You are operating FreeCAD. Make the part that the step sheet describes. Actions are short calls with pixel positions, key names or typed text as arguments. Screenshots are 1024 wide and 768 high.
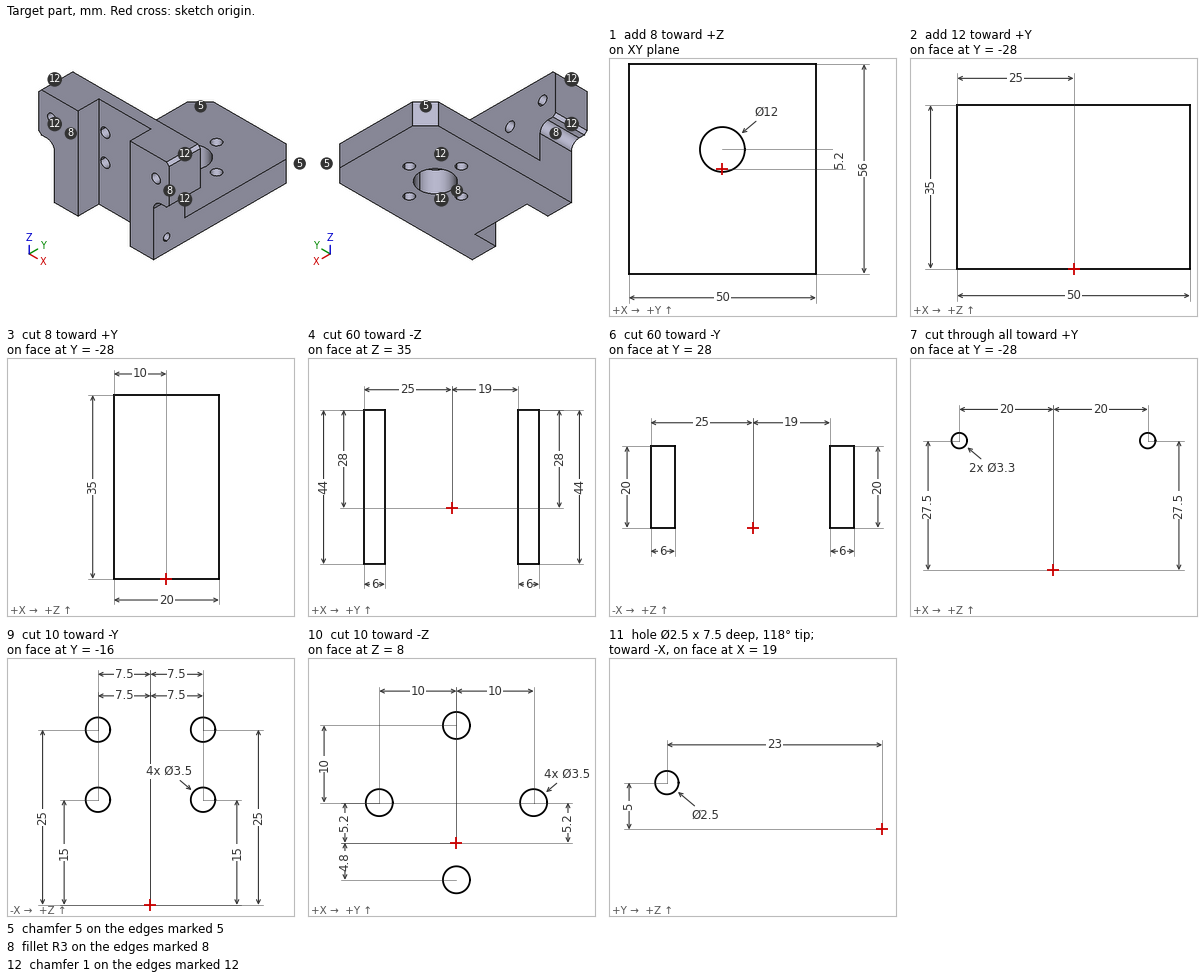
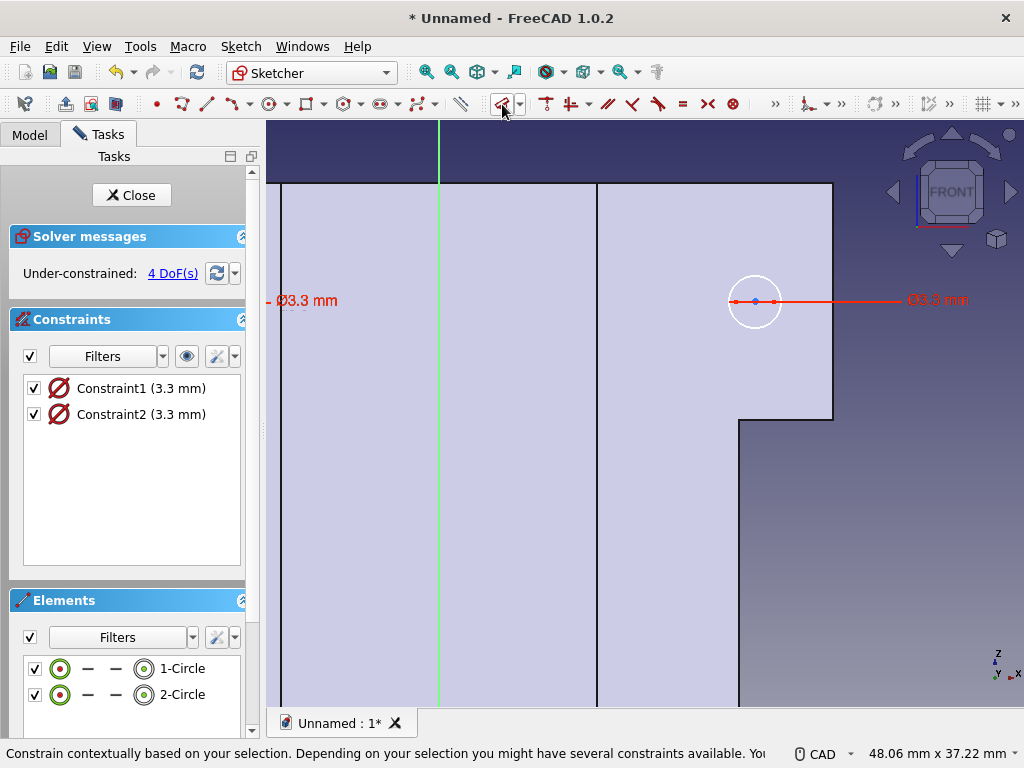
scroll(744, 302, down, 3)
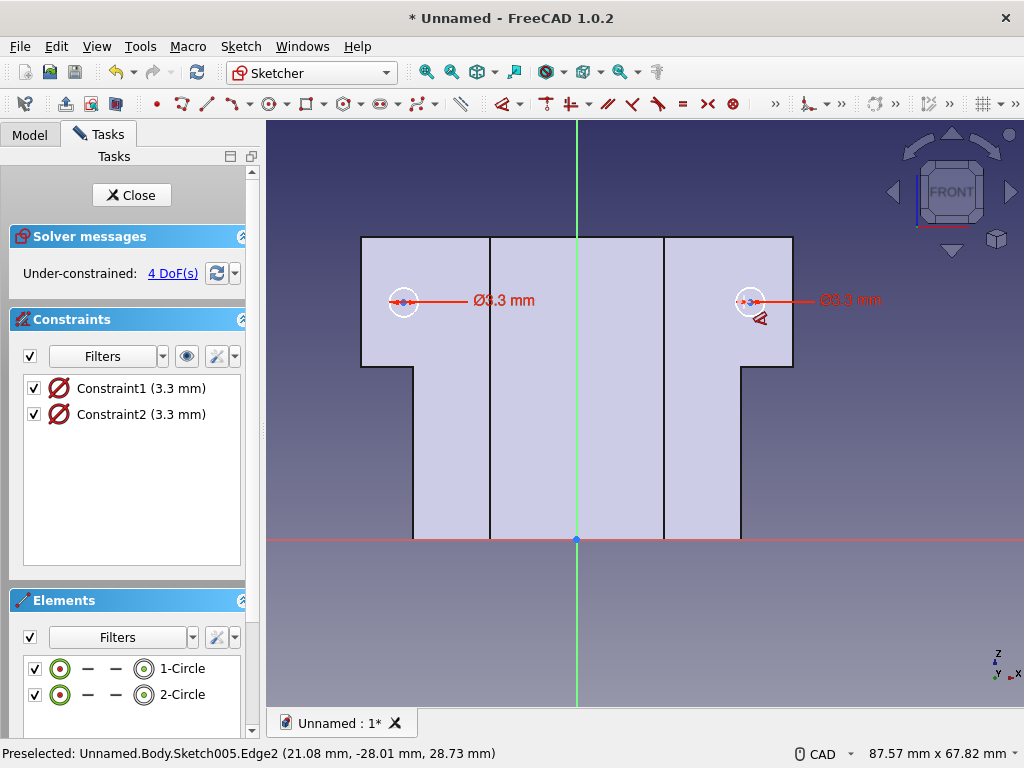
click(404, 302)
click(490, 574)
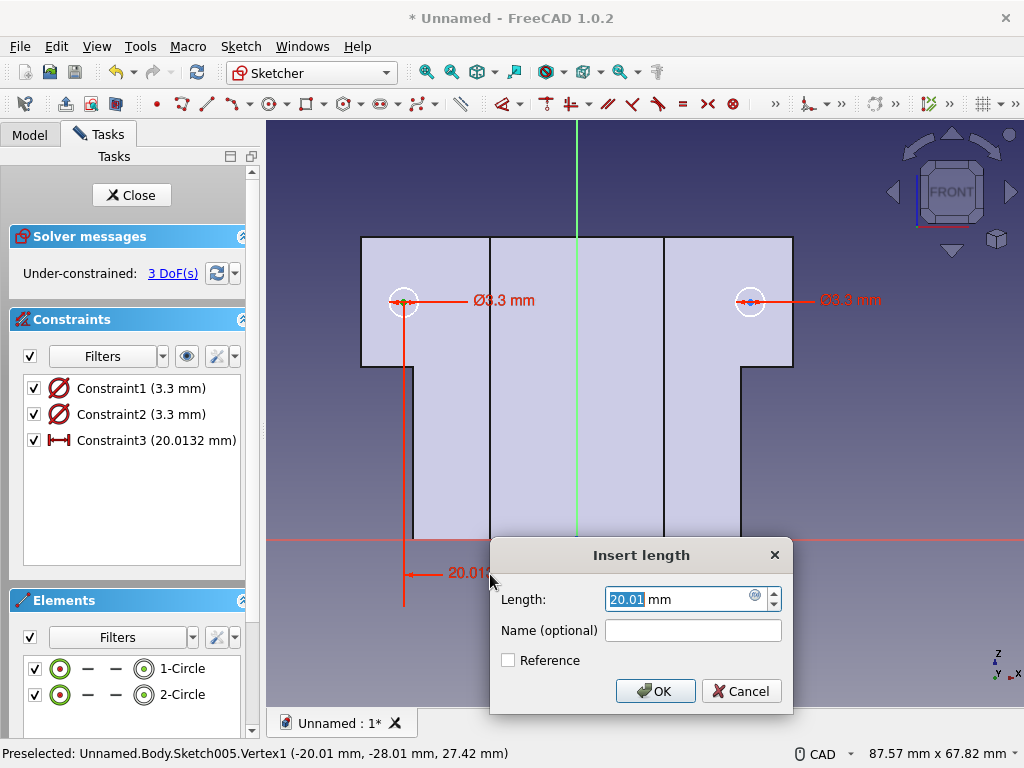
text(20)
key(Return)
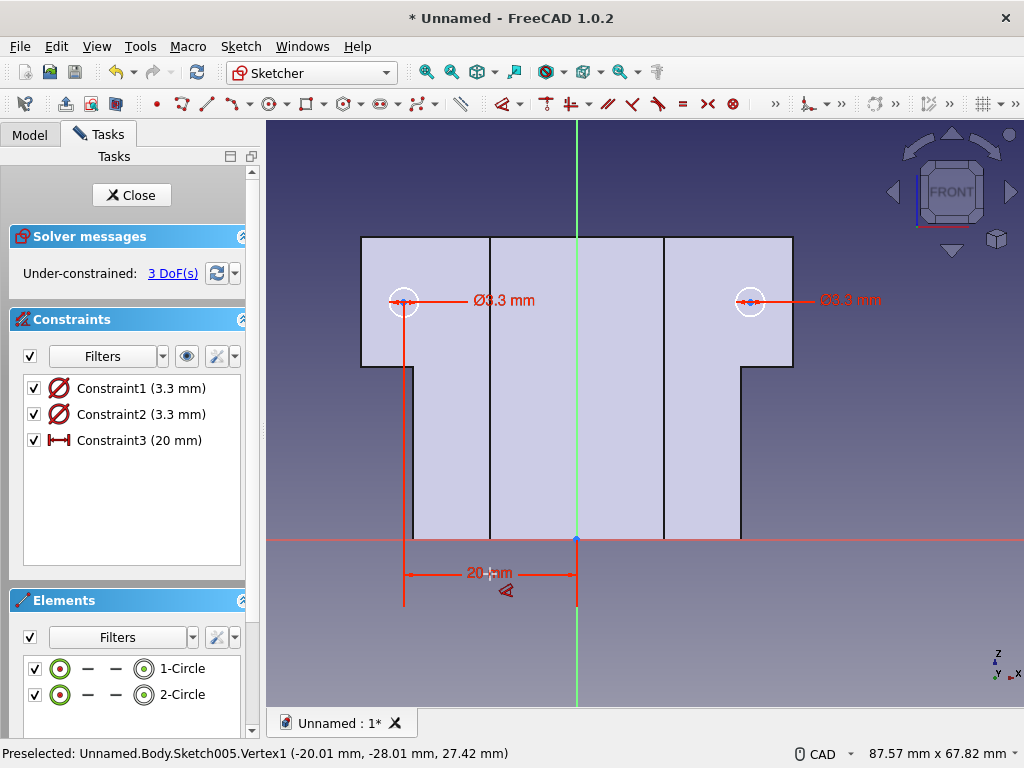
click(750, 302)
click(664, 574)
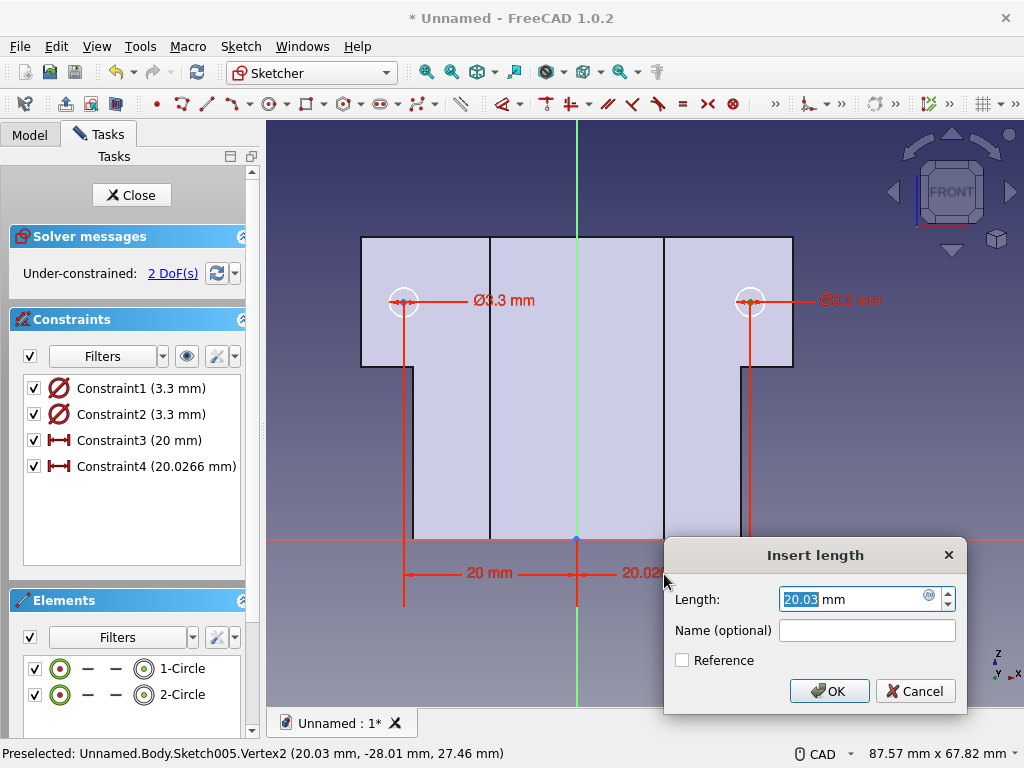
text(20)
key(Return)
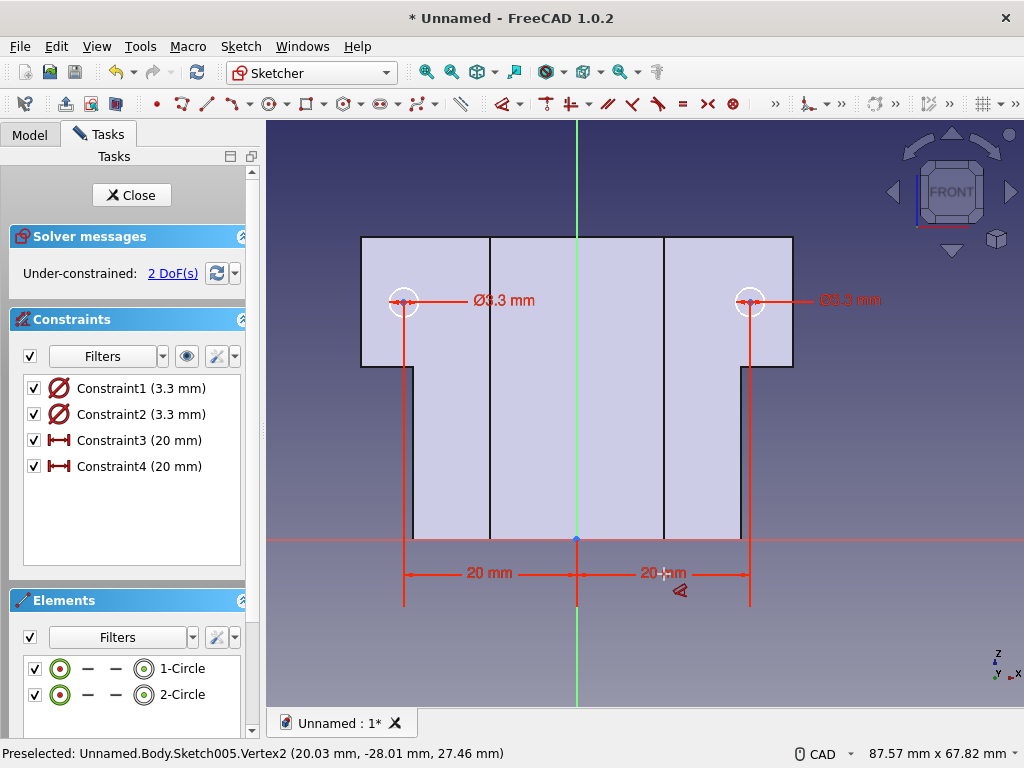
click(404, 302)
click(370, 421)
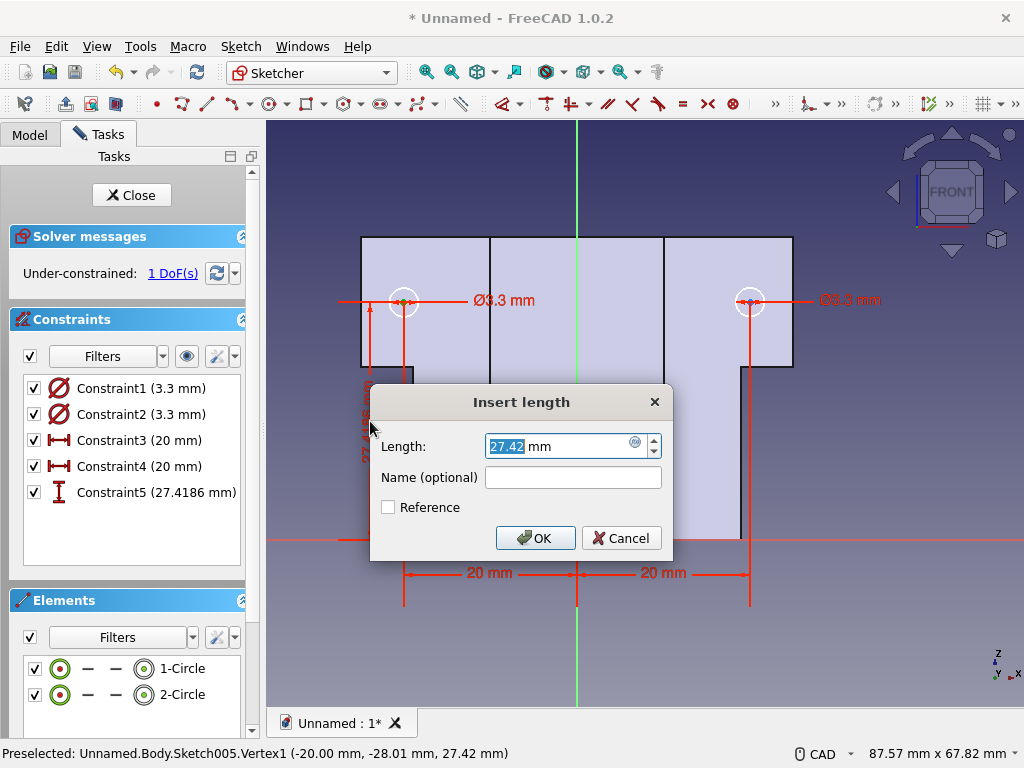
text(27.5)
key(Return)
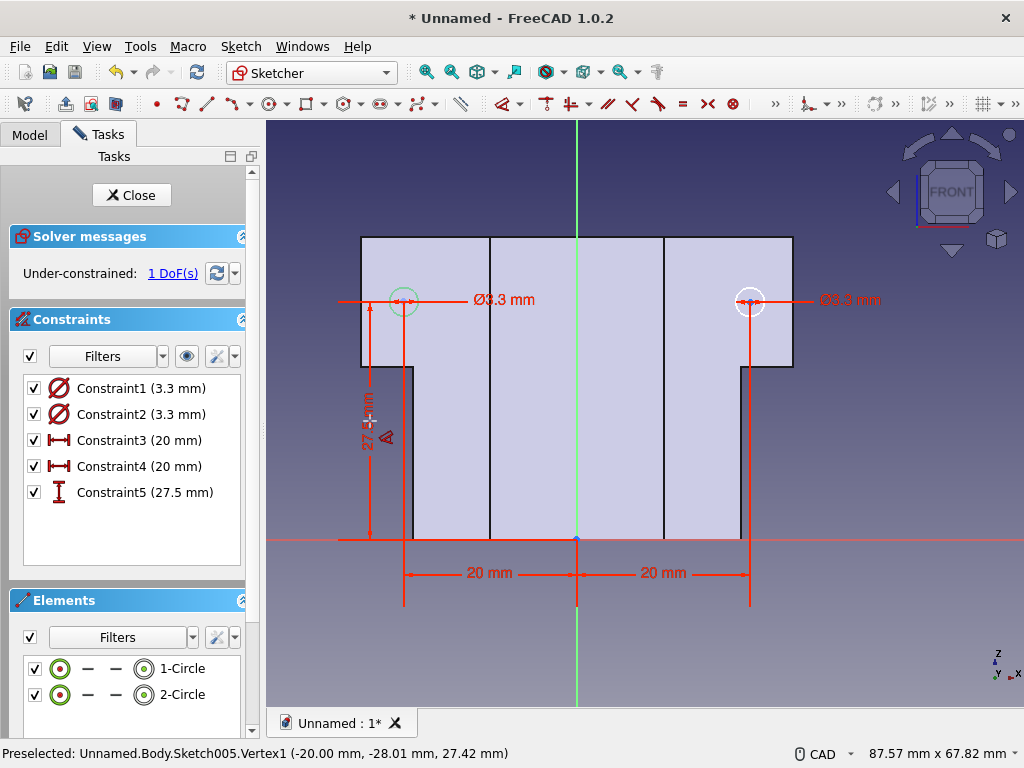
click(750, 302)
click(784, 421)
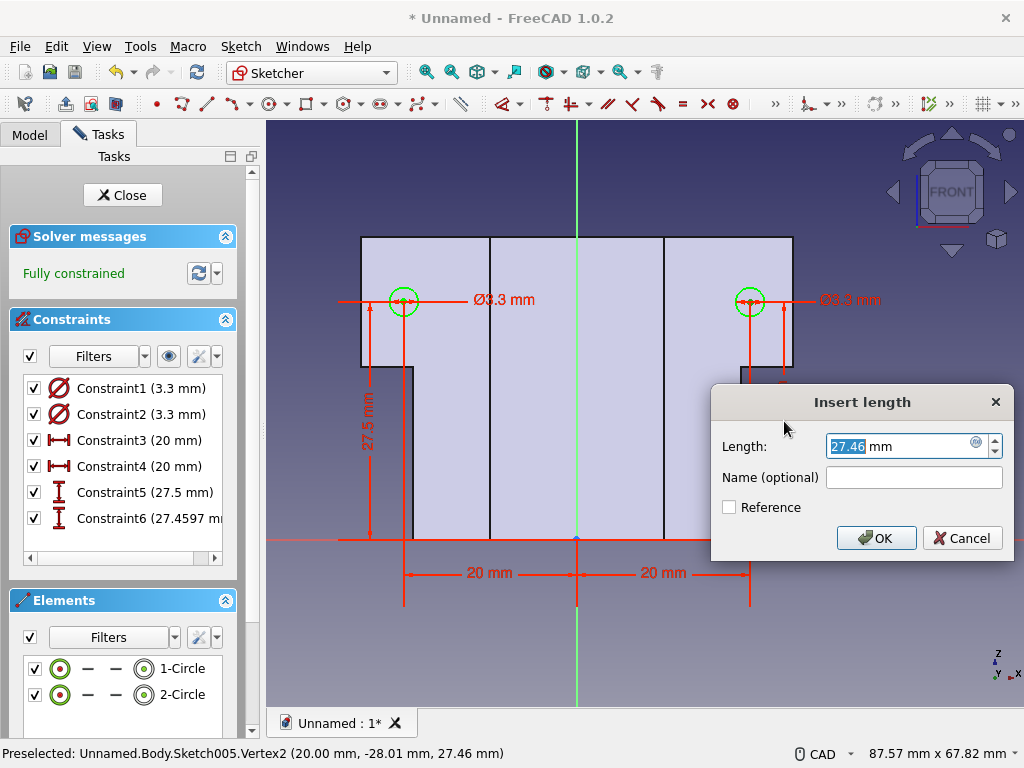
text(27.5)
key(Return)
key(Escape)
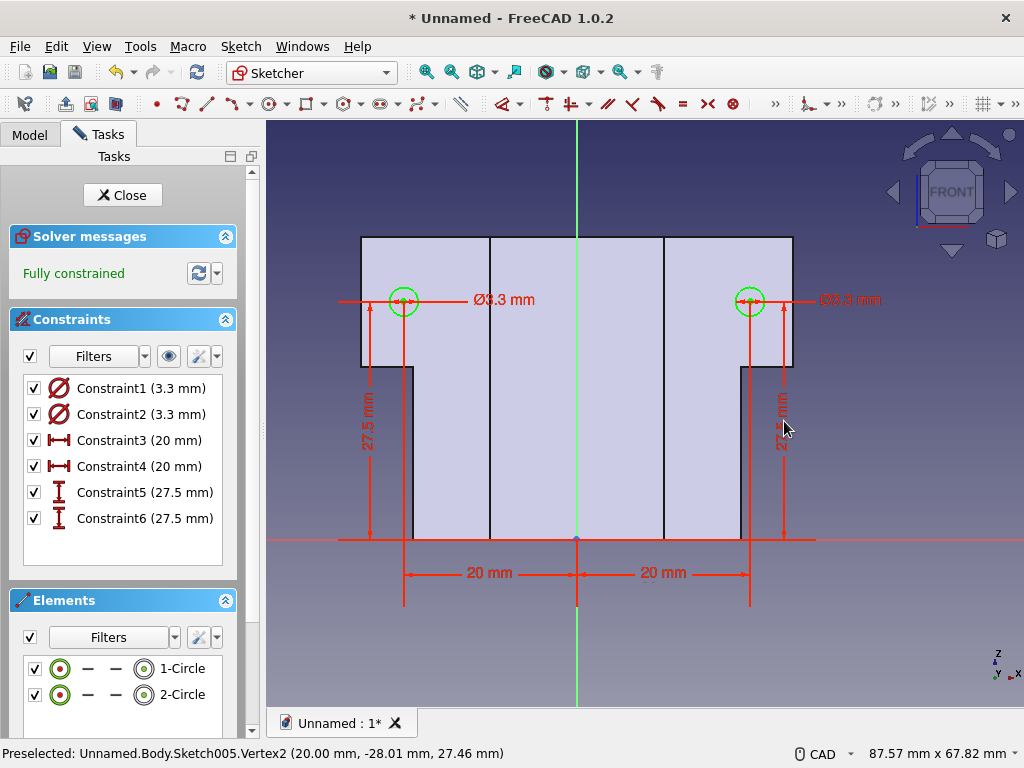
click(123, 195)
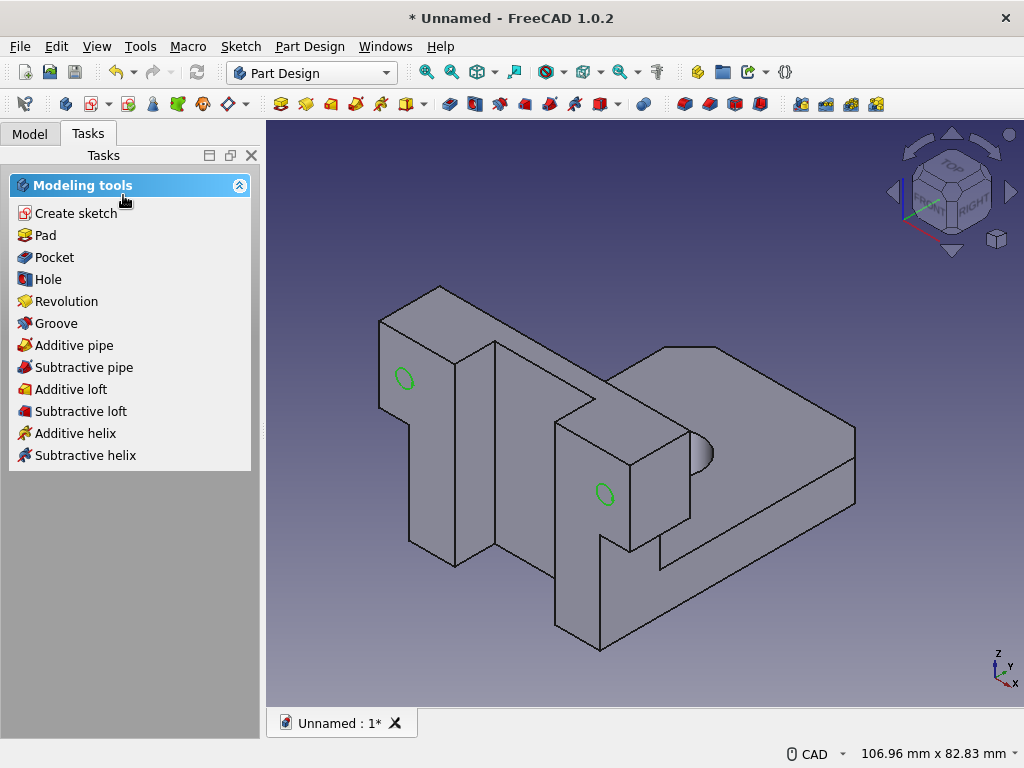
click(450, 104)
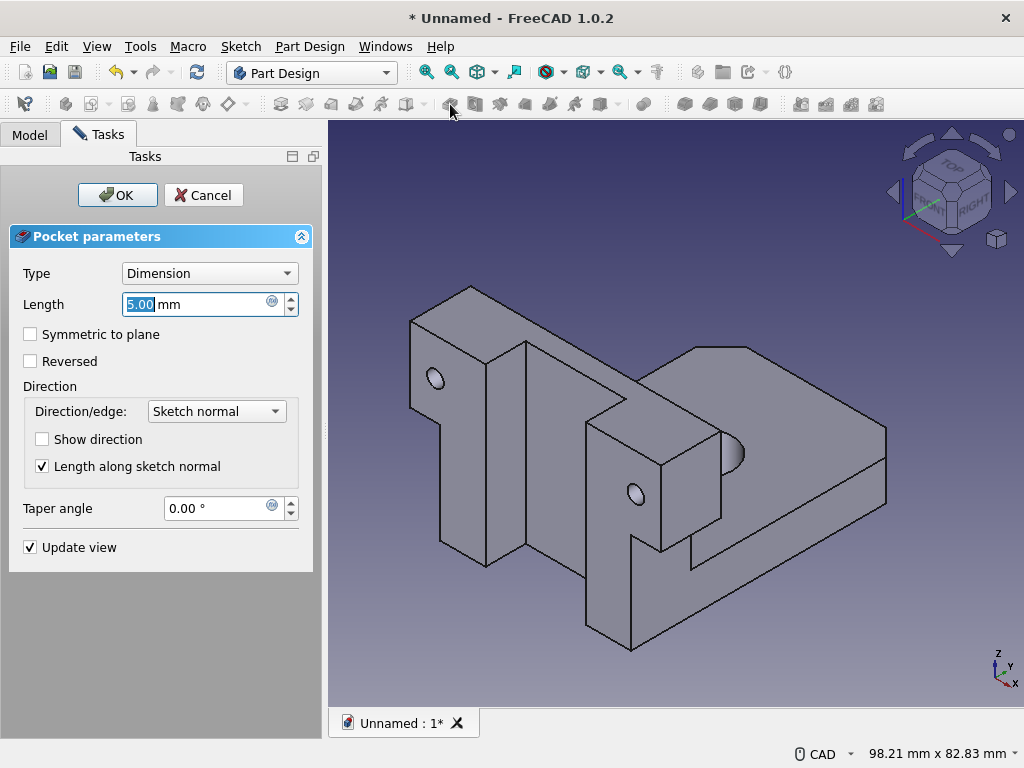
click(210, 274)